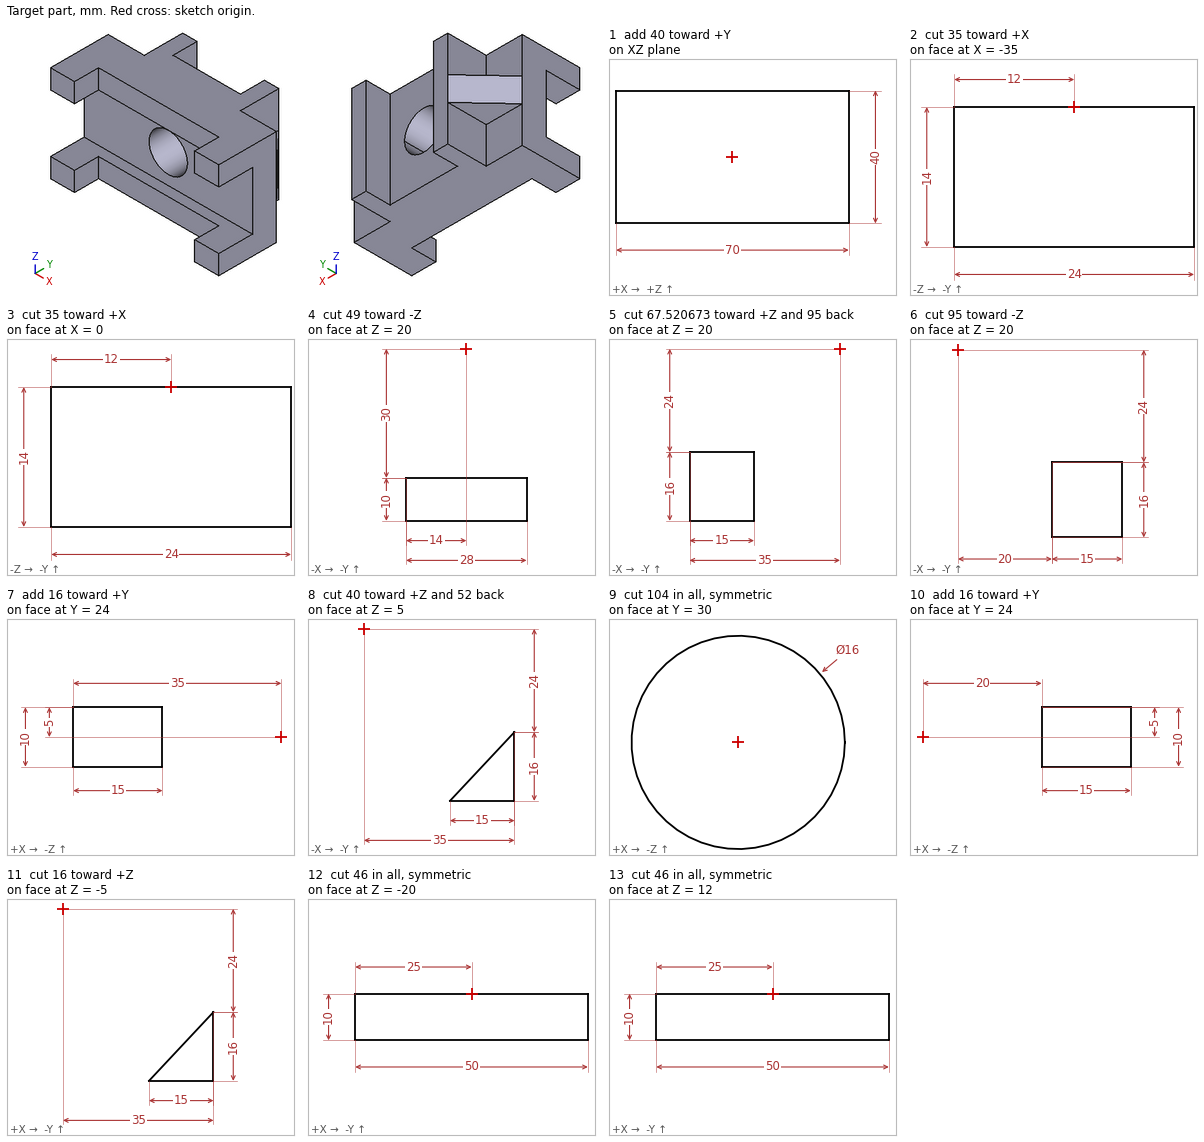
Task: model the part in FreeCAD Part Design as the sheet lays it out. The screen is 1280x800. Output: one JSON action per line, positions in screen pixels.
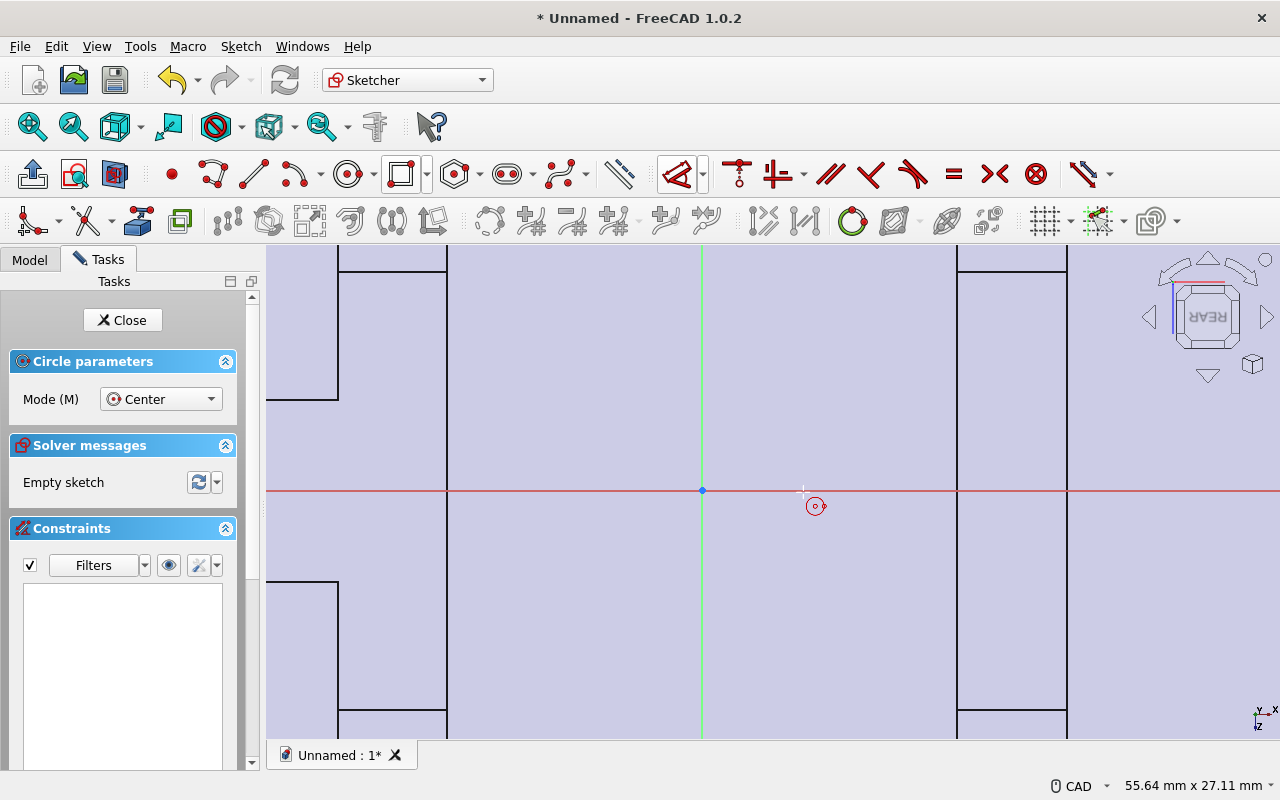
{"action": "left_click", "coordinate": [702, 491]}
{"action": "left_click", "coordinate": [805, 388]}
{"action": "key", "text": "Escape"}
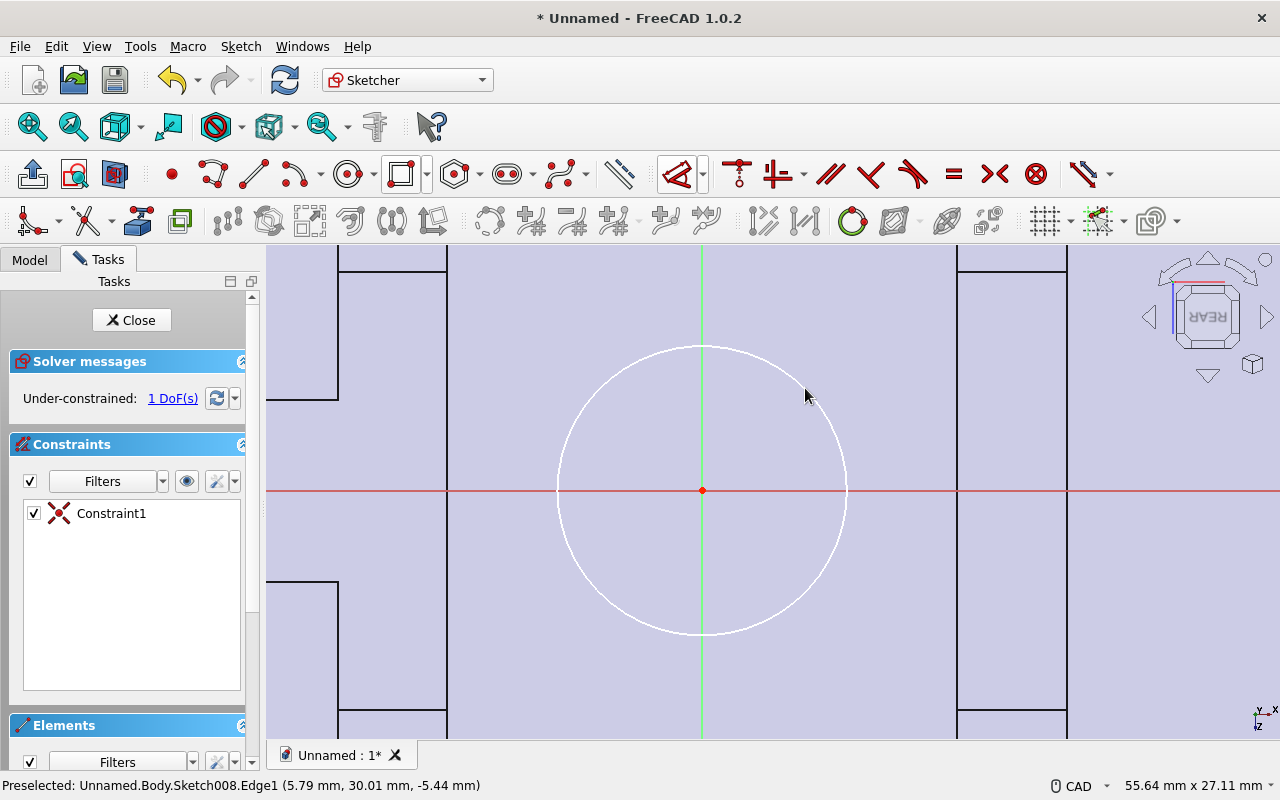
{"action": "left_click", "coordinate": [804, 388]}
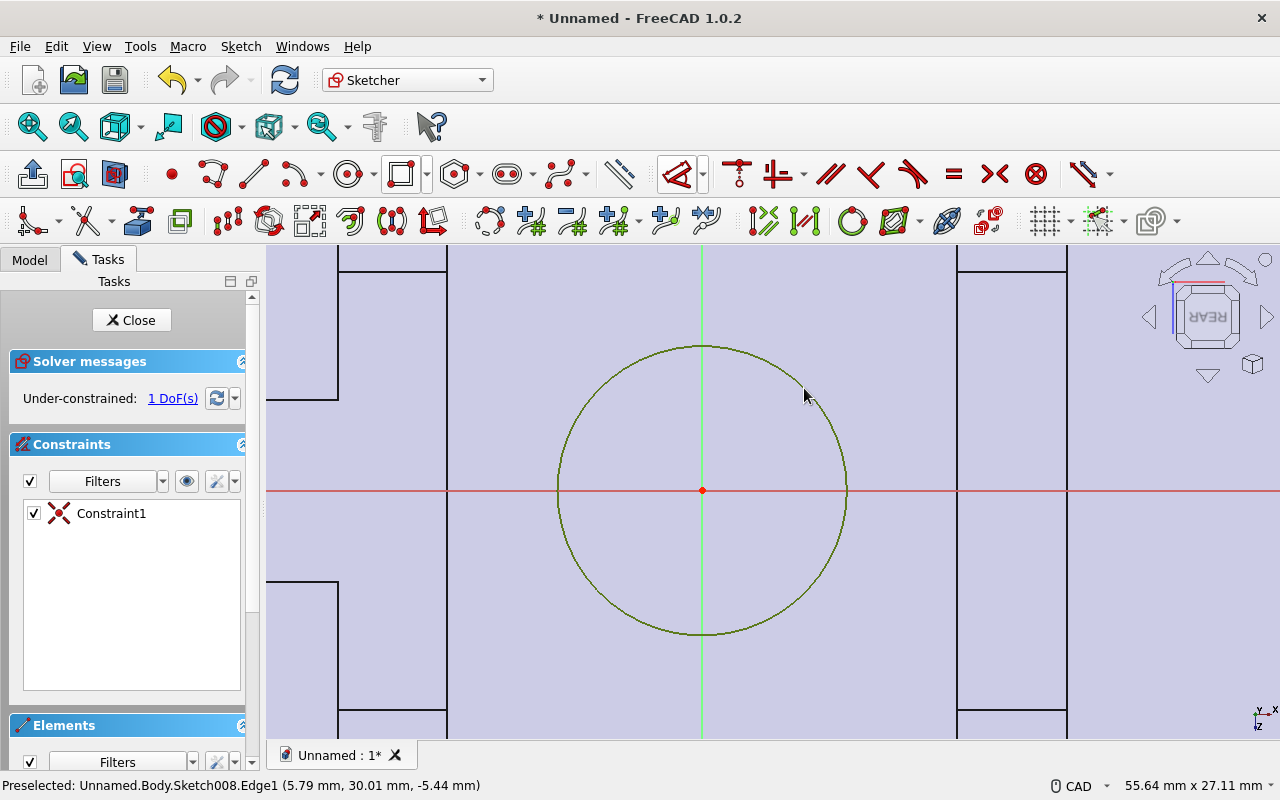
{"action": "key", "text": "k o"}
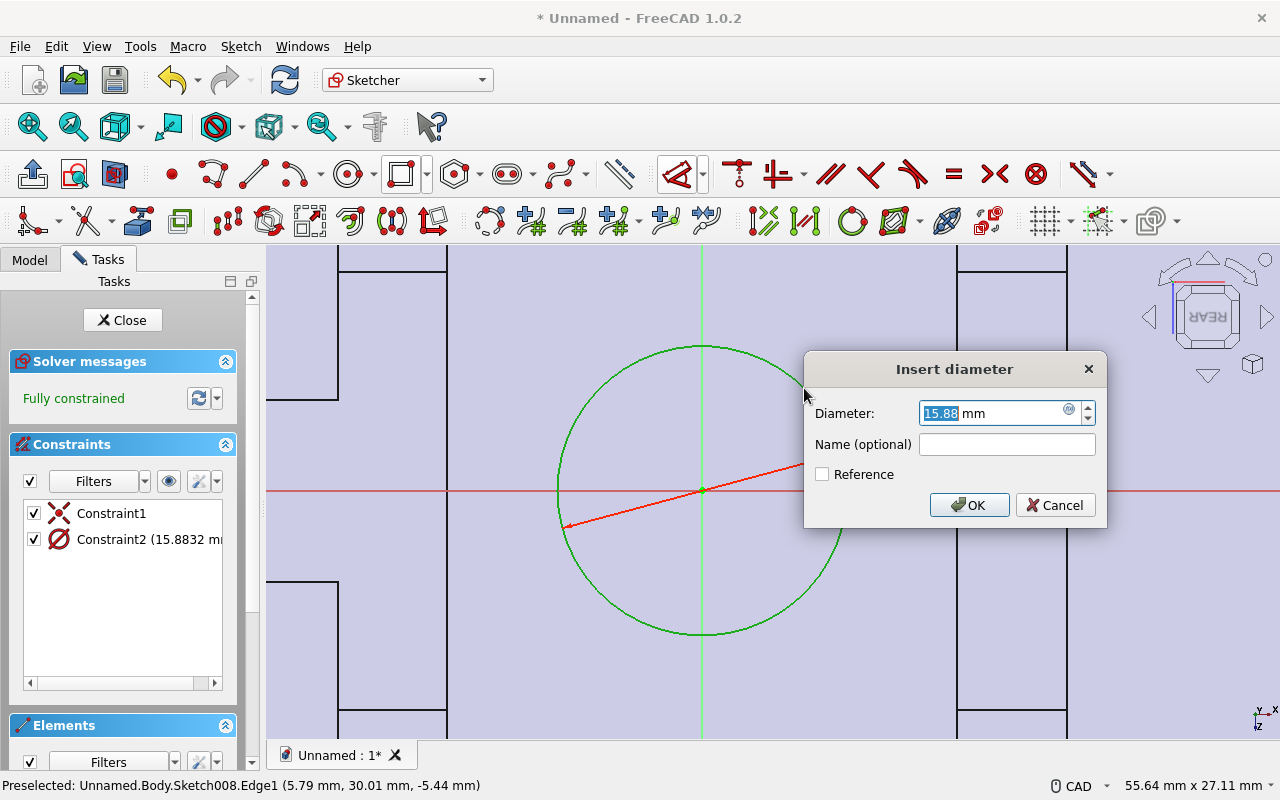
{"action": "type", "text": "16"}
{"action": "key", "text": "Return"}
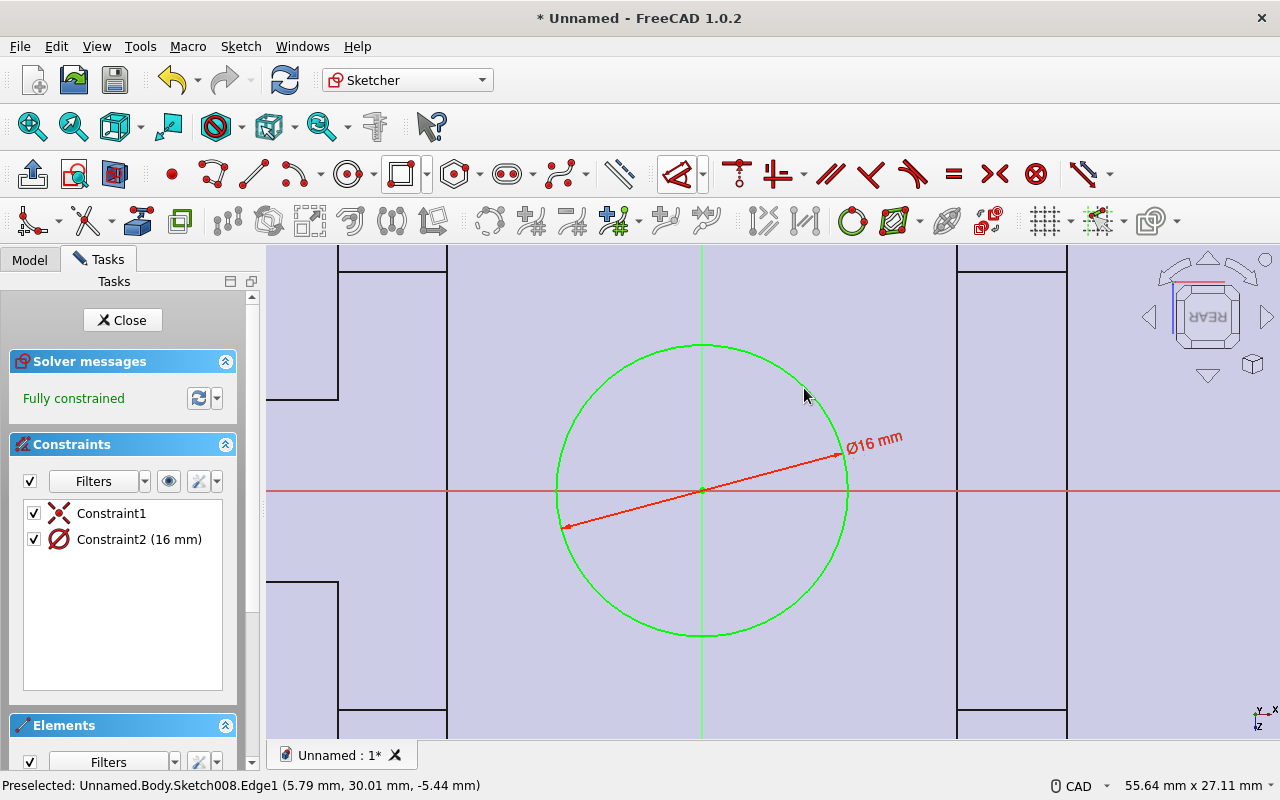
{"action": "left_click", "coordinate": [123, 320]}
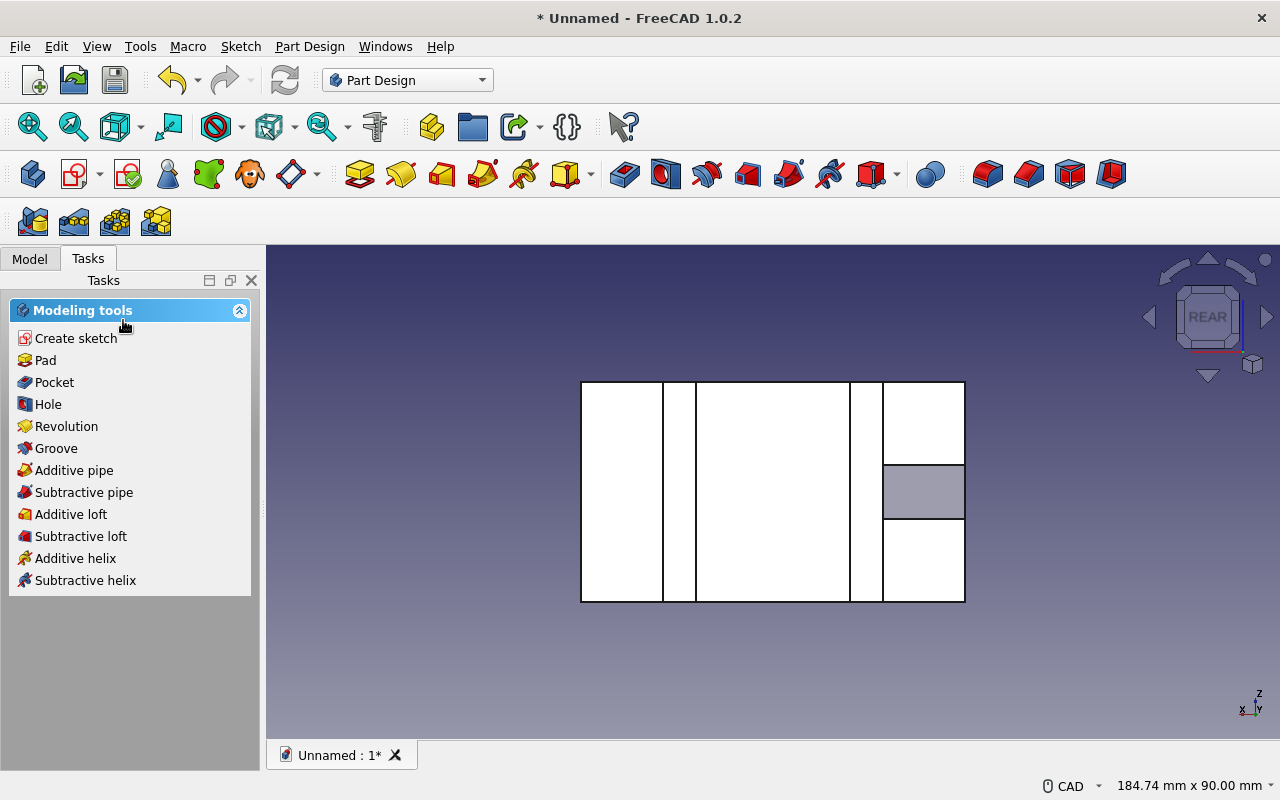
{"action": "left_click", "coordinate": [625, 174]}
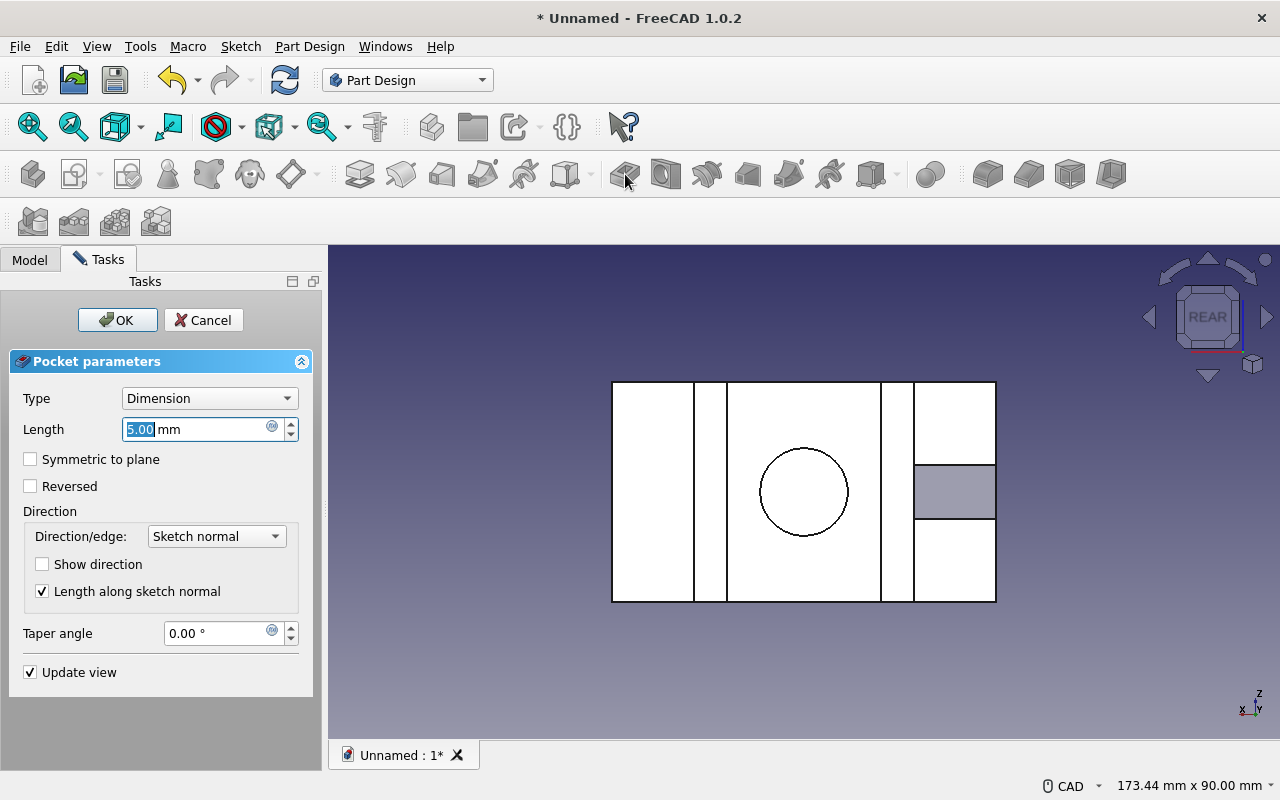
{"action": "type", "text": "104"}
{"action": "key", "text": "Tab"}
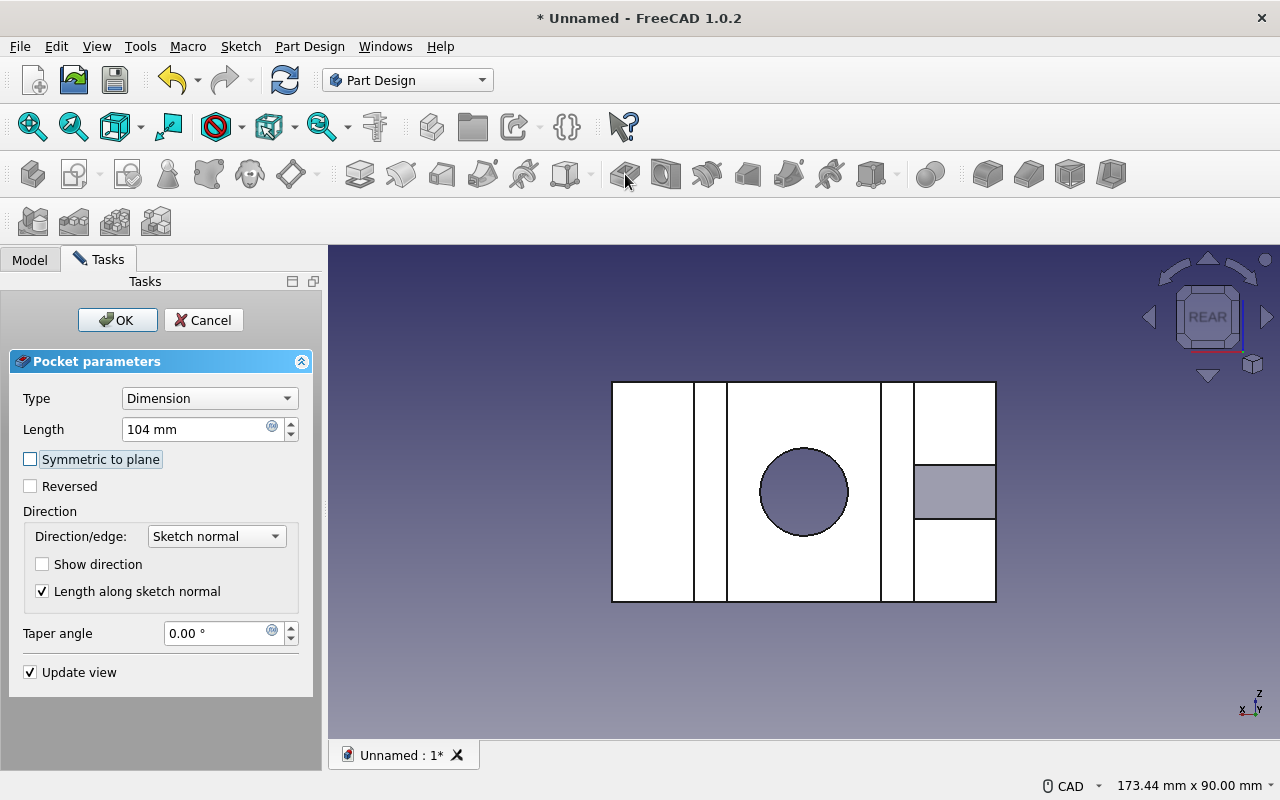
{"action": "left_click", "coordinate": [31, 459]}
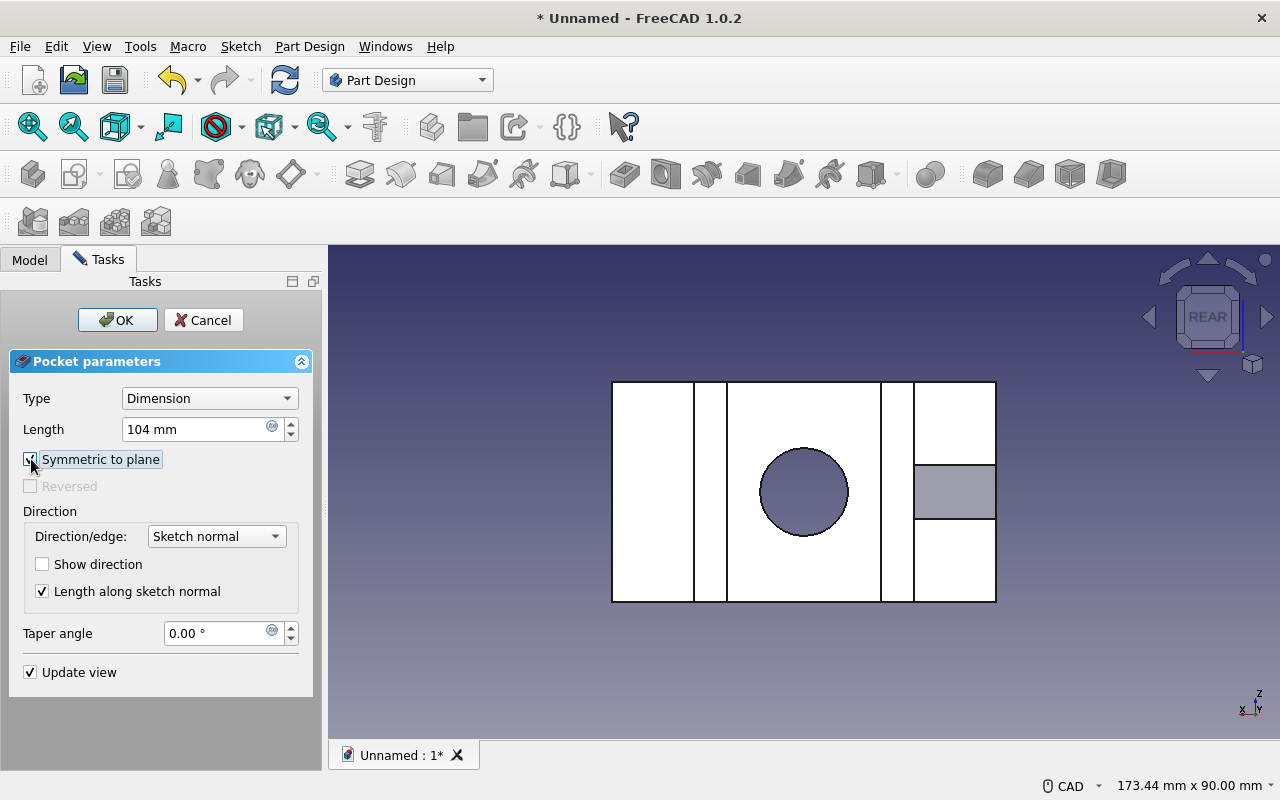
{"action": "left_click", "coordinate": [118, 320]}